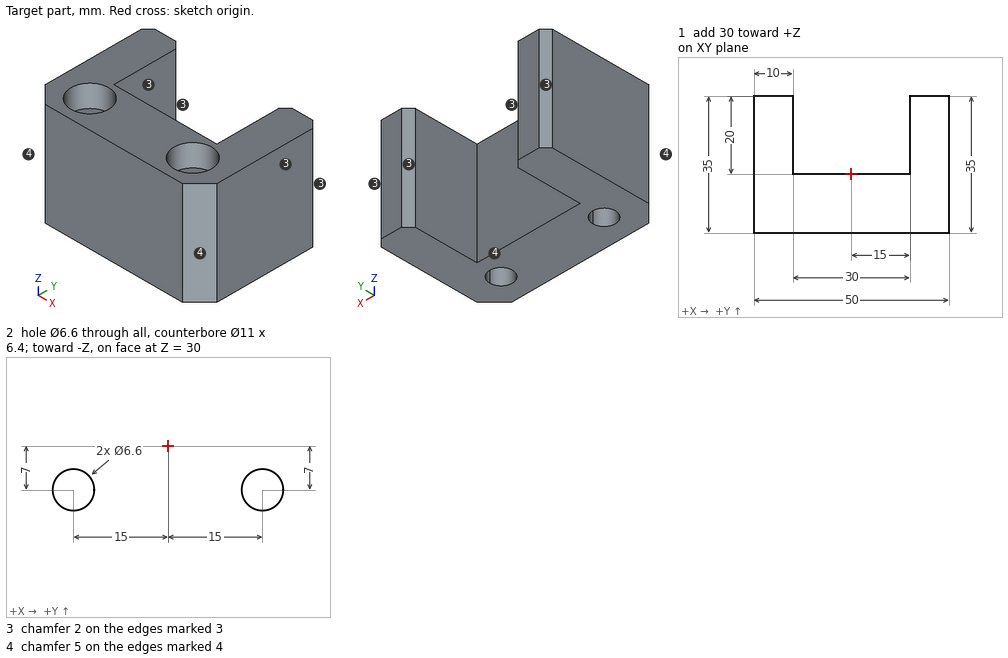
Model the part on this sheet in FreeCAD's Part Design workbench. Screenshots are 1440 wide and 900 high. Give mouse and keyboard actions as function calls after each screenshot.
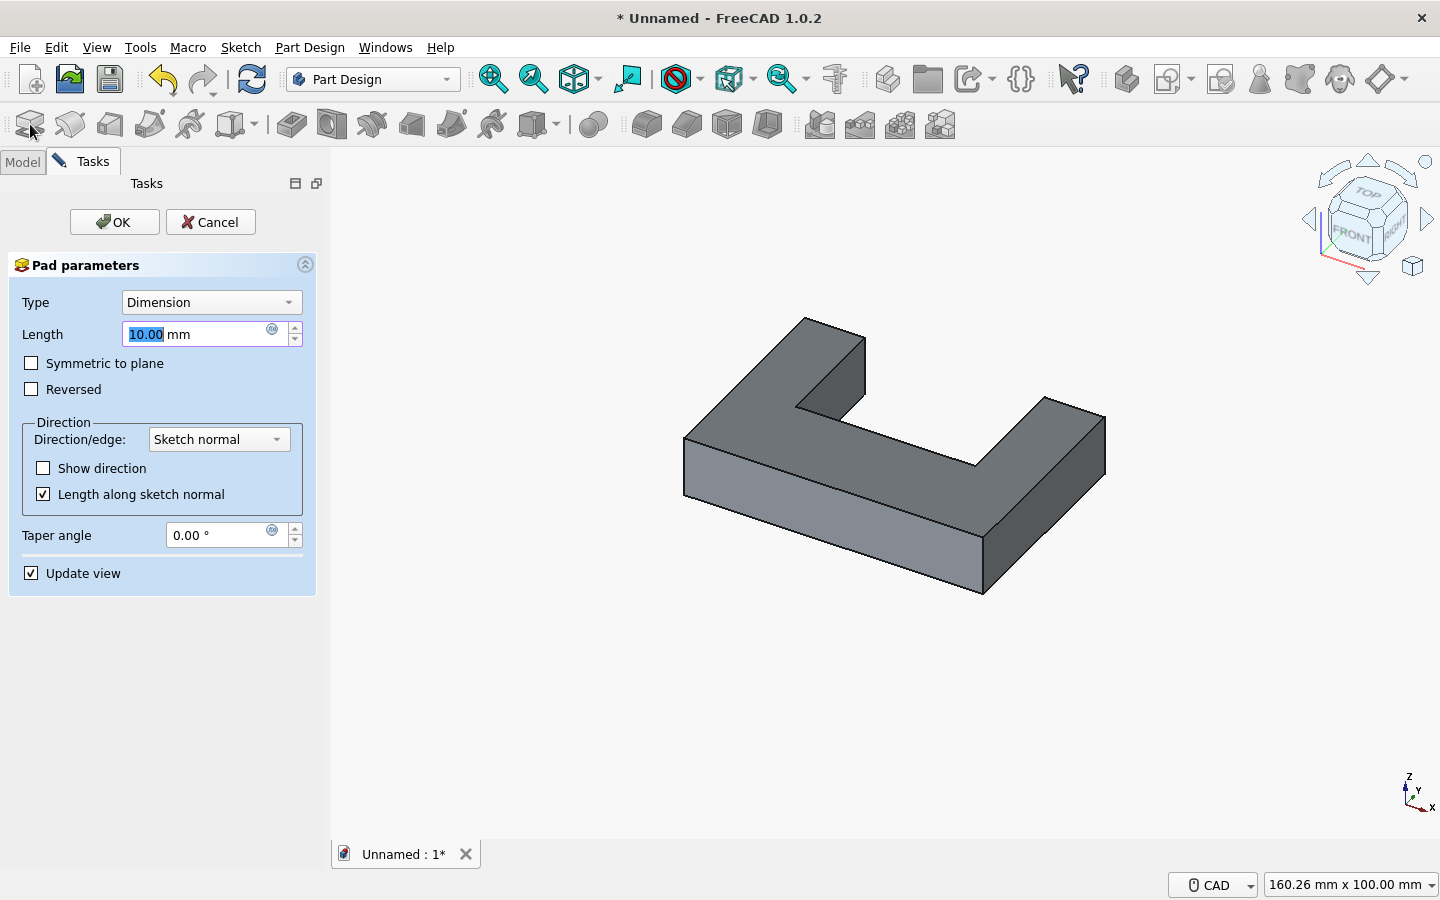
text(30)
key(Tab)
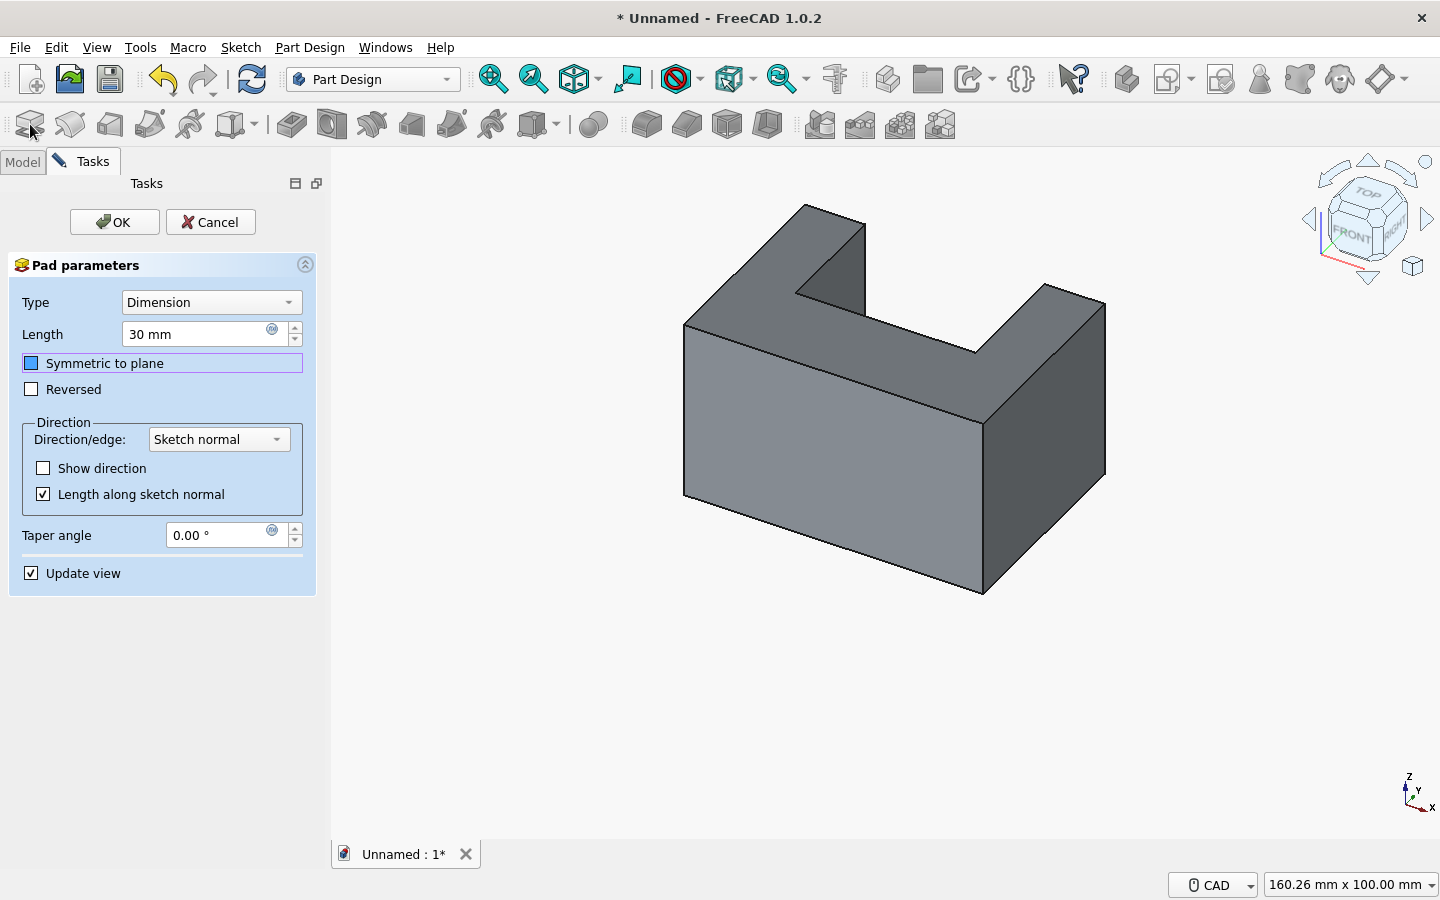
click(115, 222)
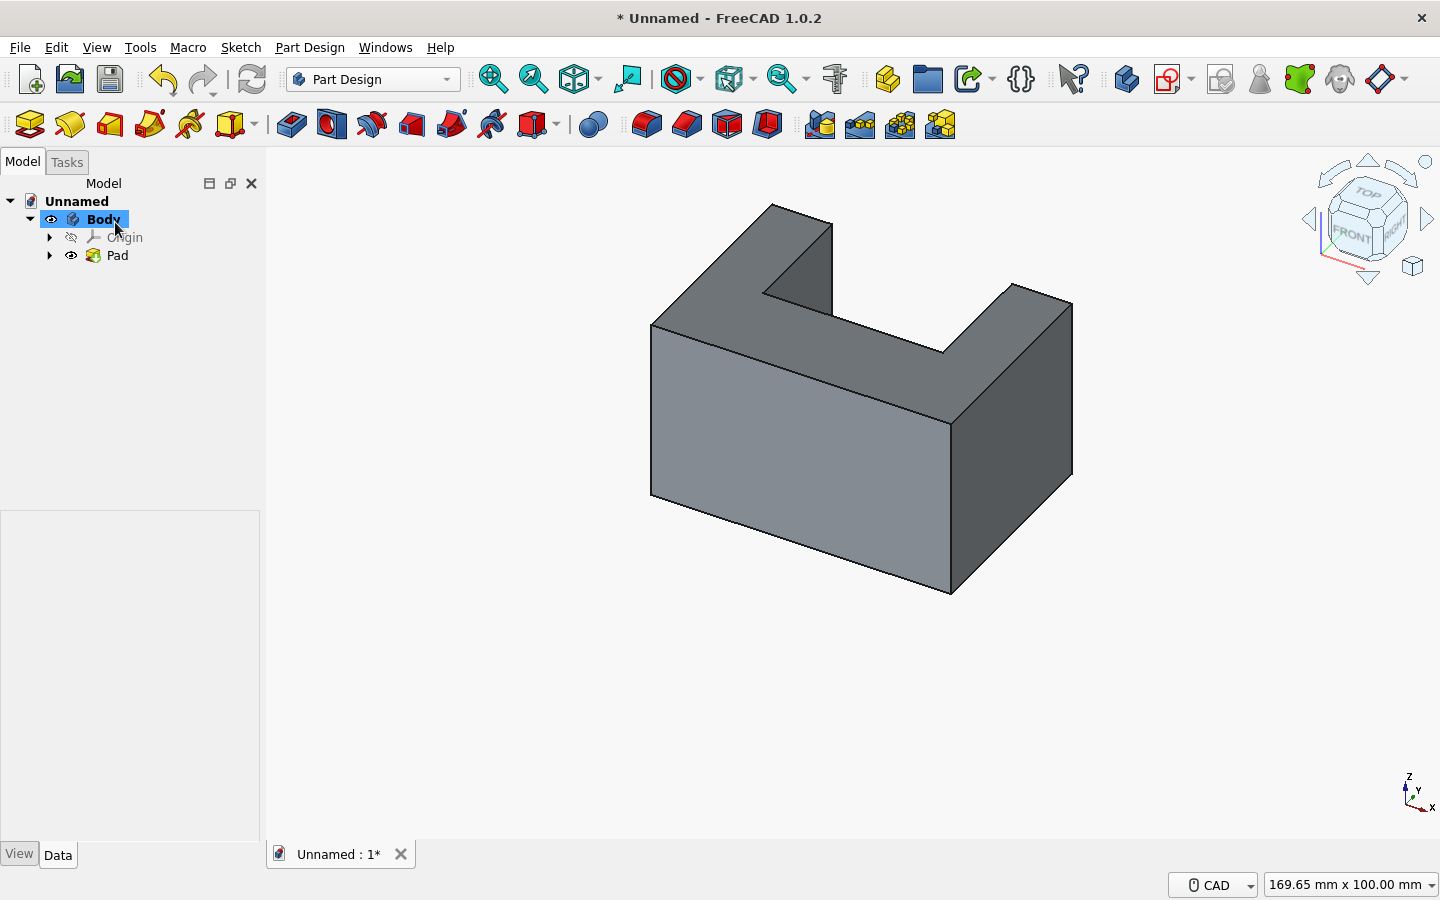
click(913, 376)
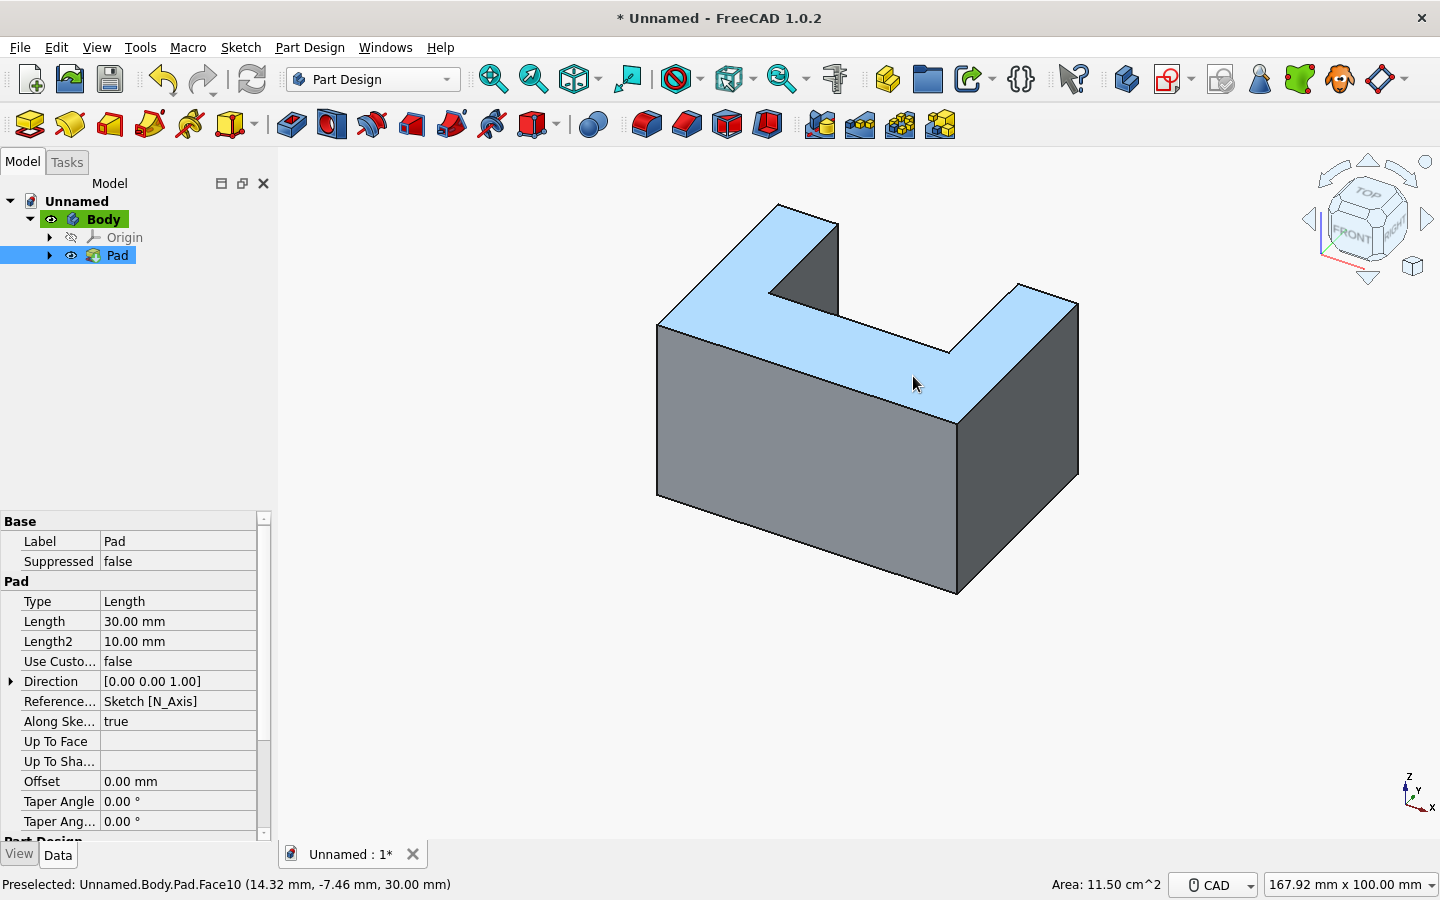
click(1168, 80)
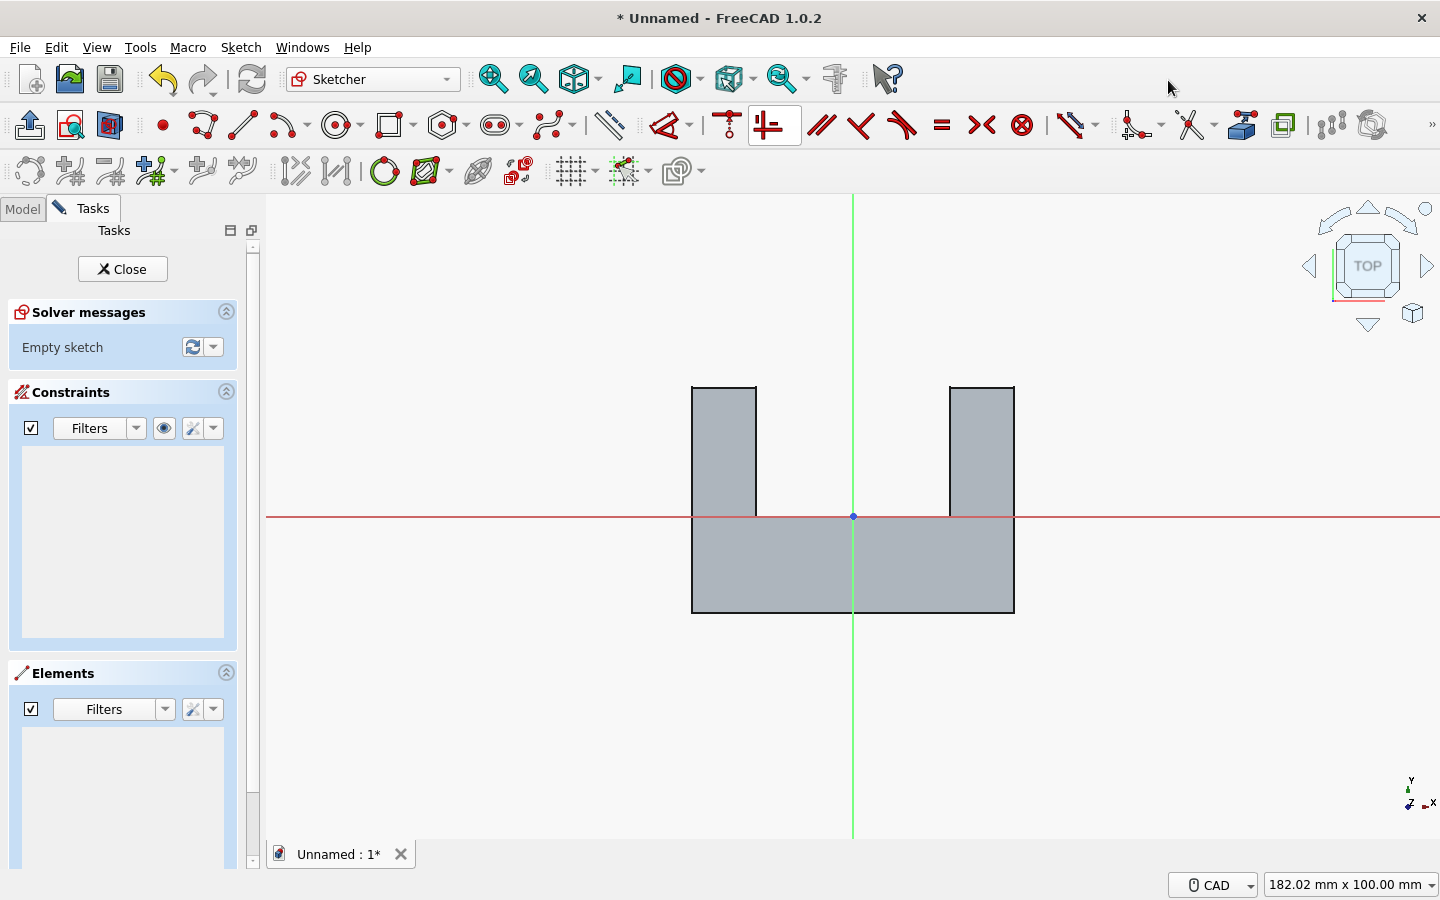
scroll(893, 569, up, 5)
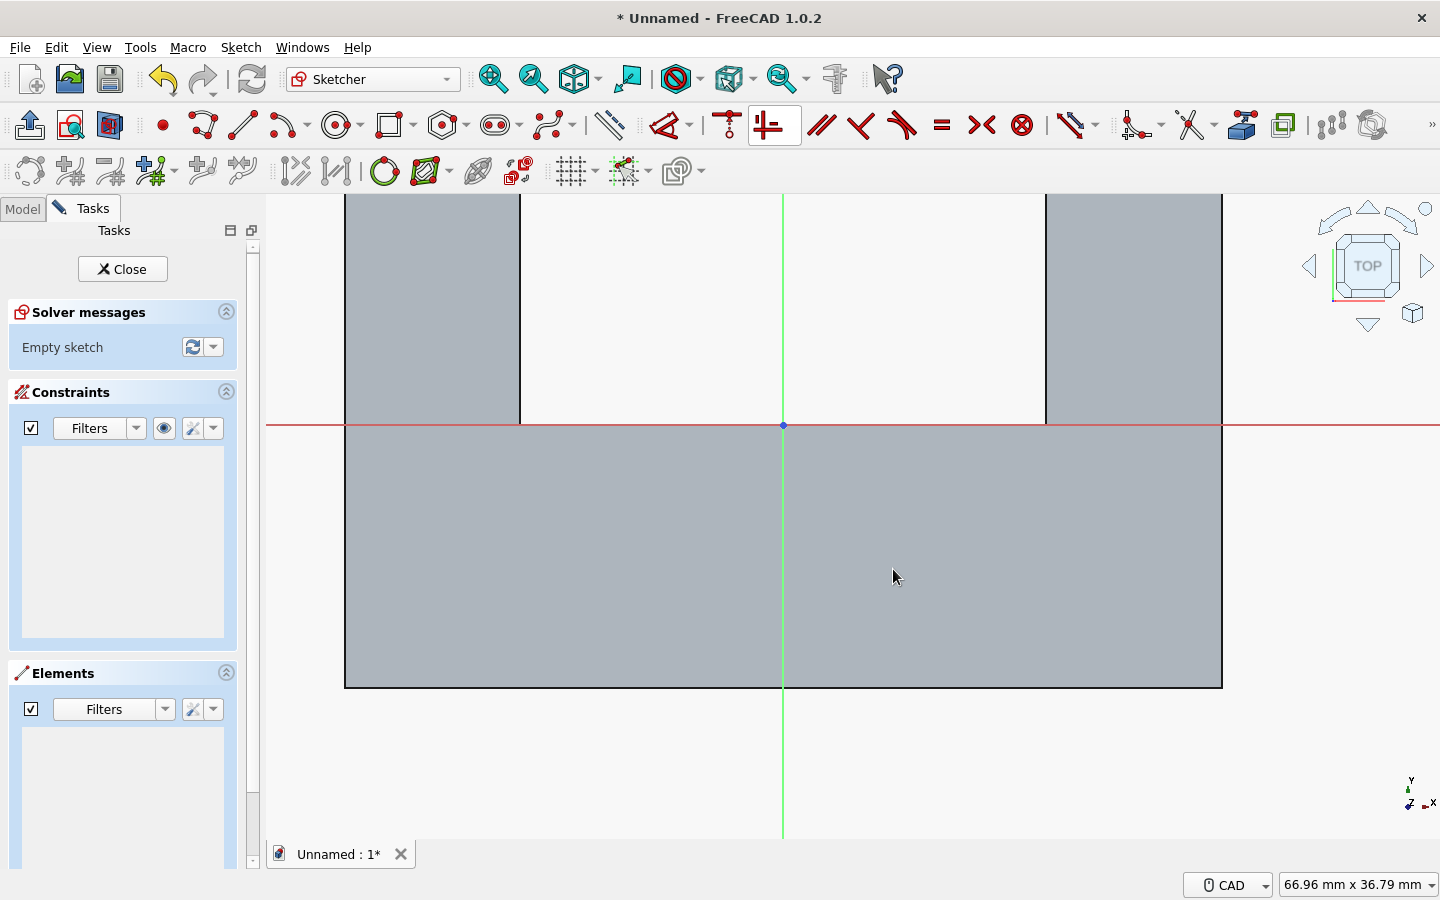
click(336, 126)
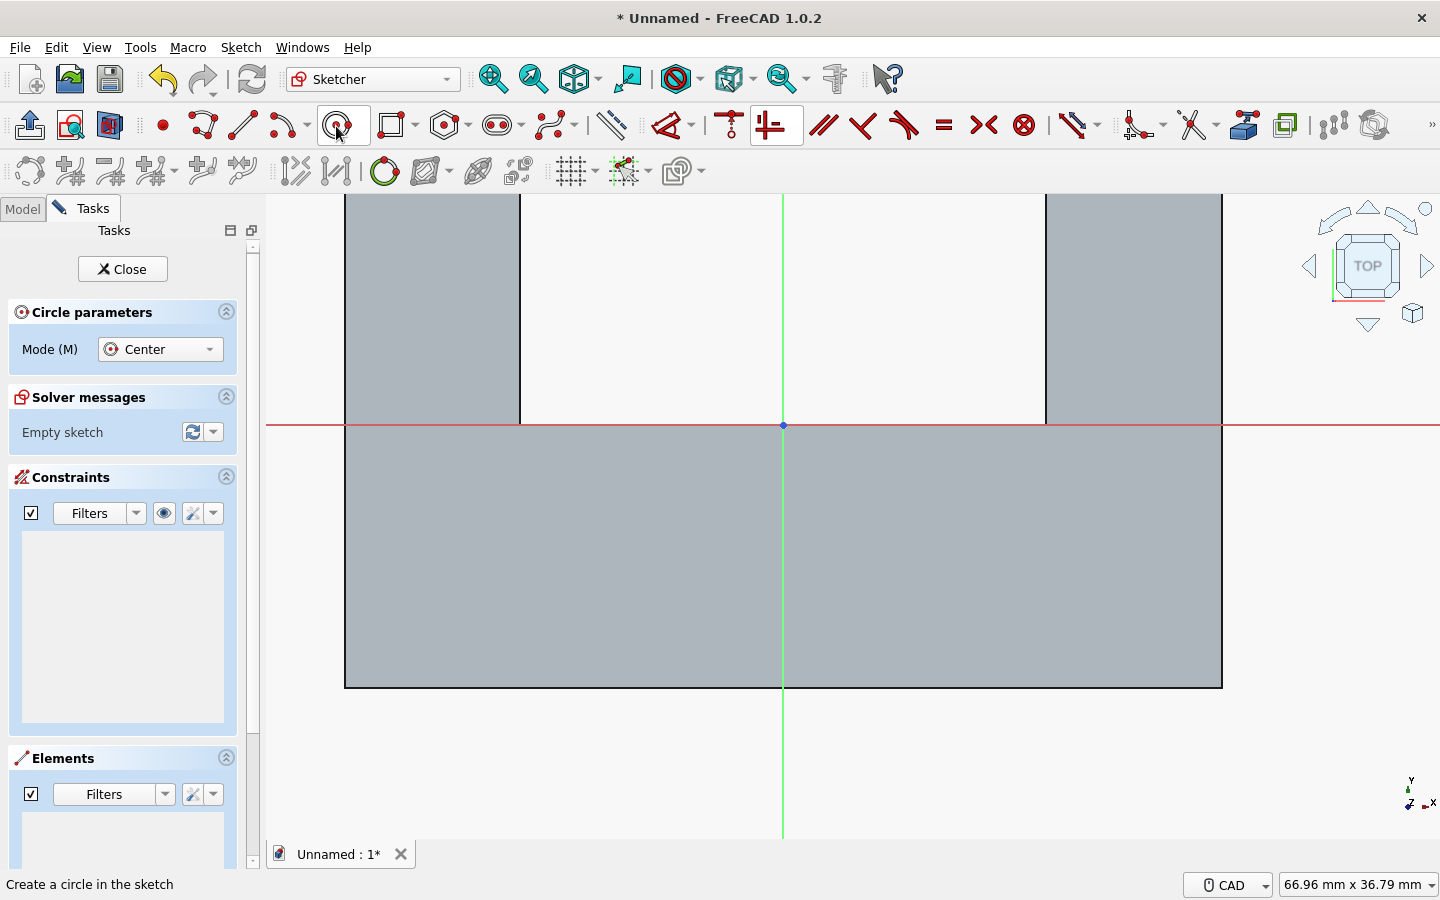
click(520, 548)
click(561, 507)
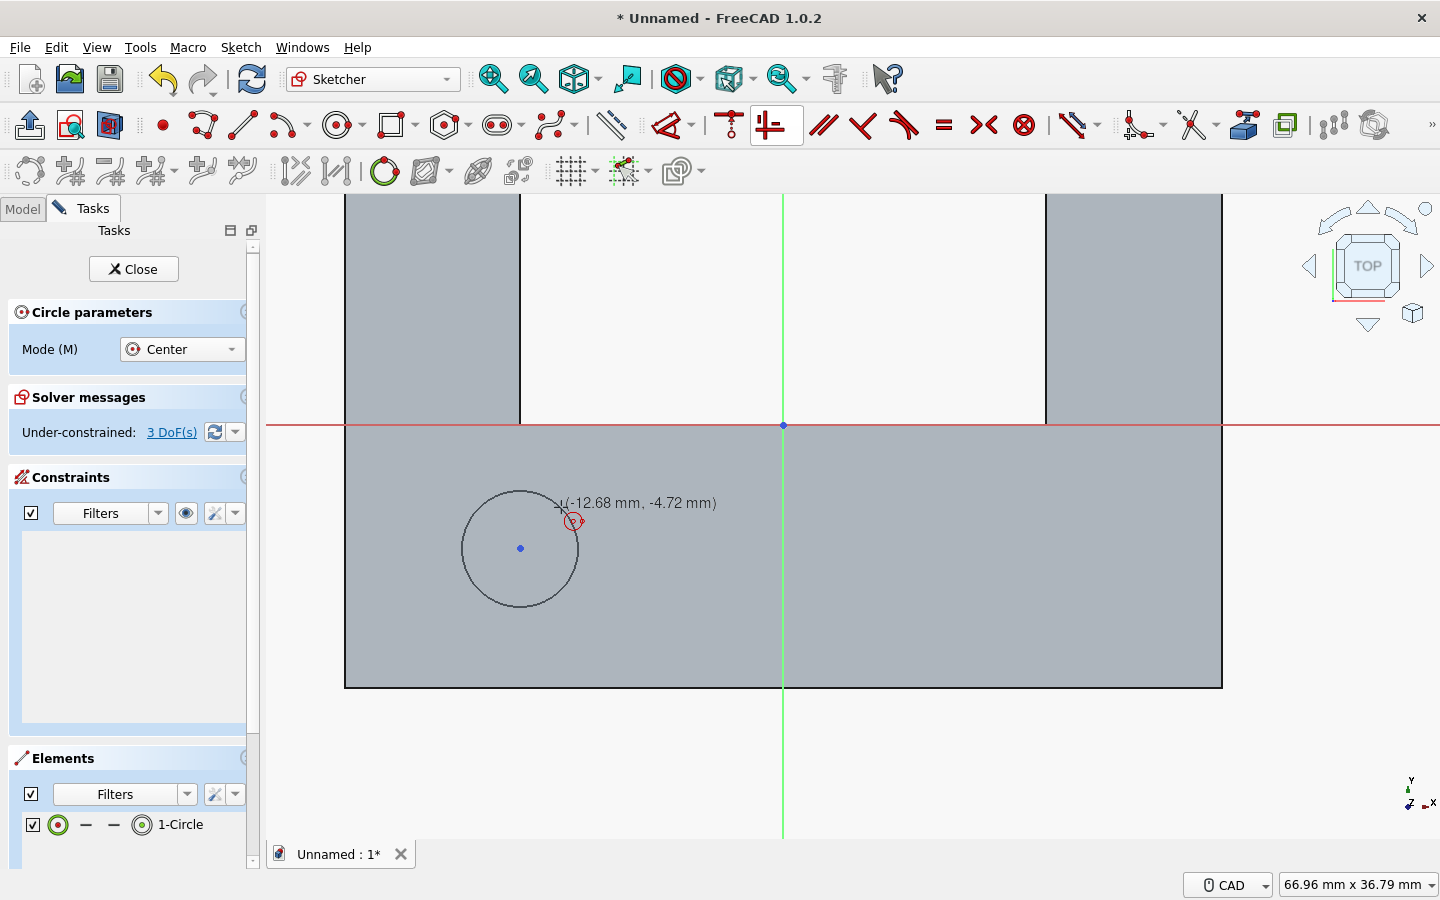
click(1046, 548)
click(1087, 507)
key(Escape)